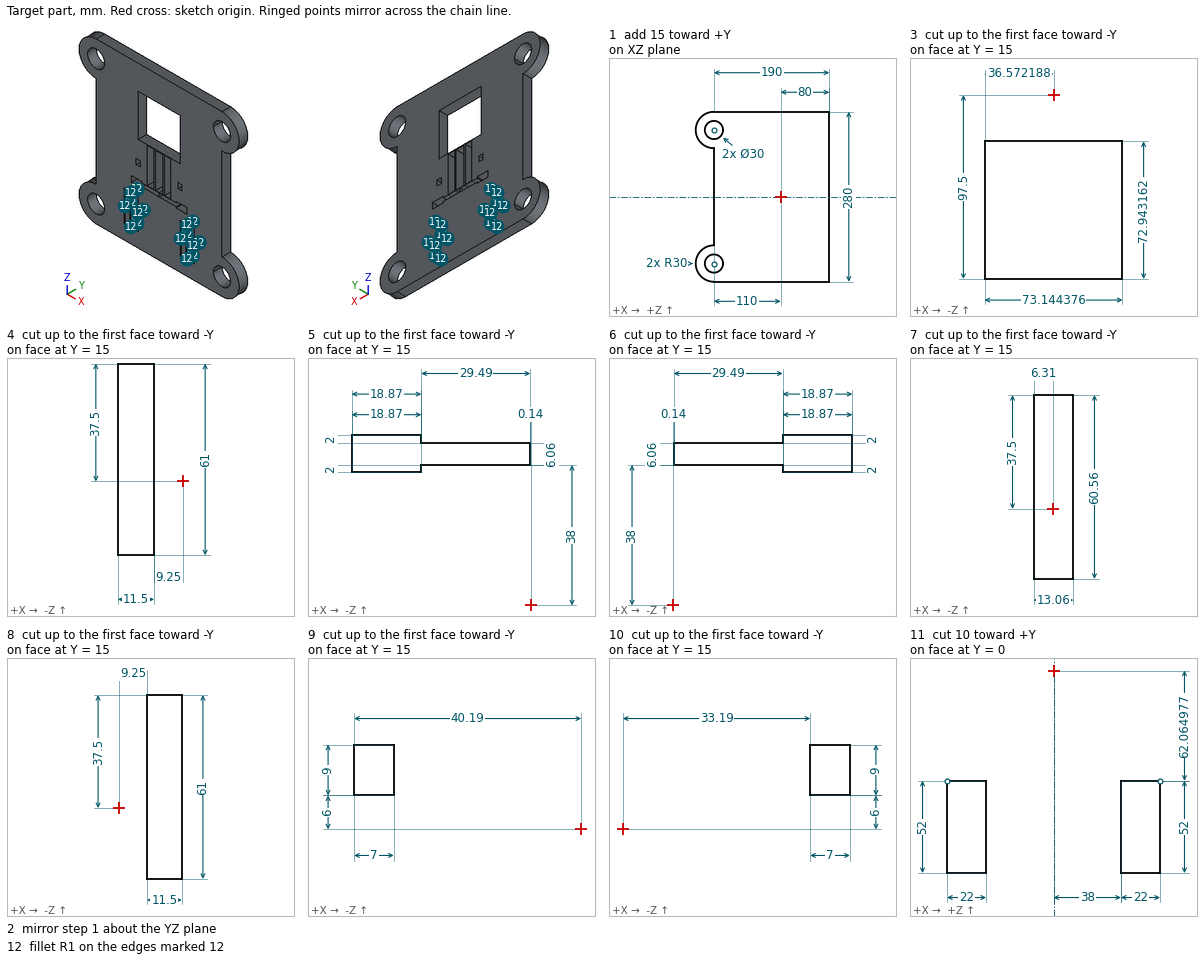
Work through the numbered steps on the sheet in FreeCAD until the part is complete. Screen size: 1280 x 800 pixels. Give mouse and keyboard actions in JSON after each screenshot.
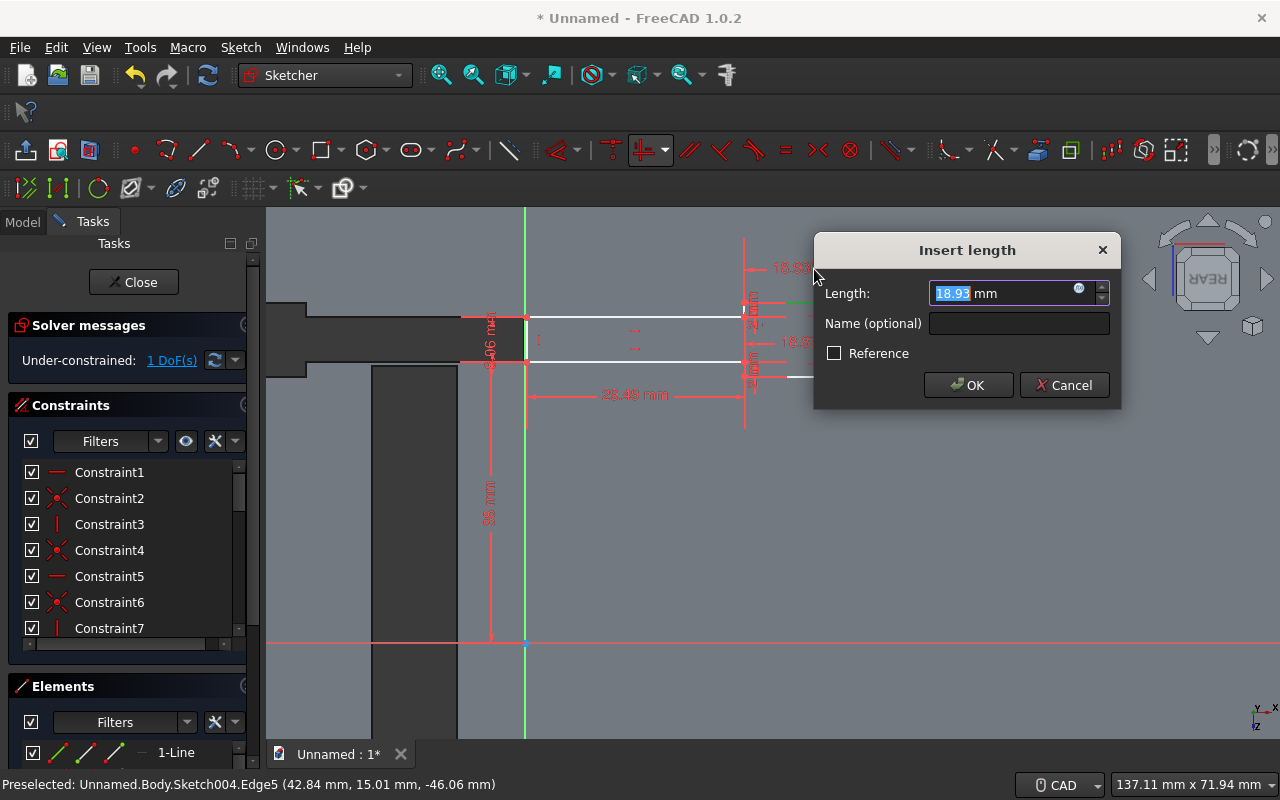
{"action": "type", "text": "18.87"}
{"action": "key", "text": "Return"}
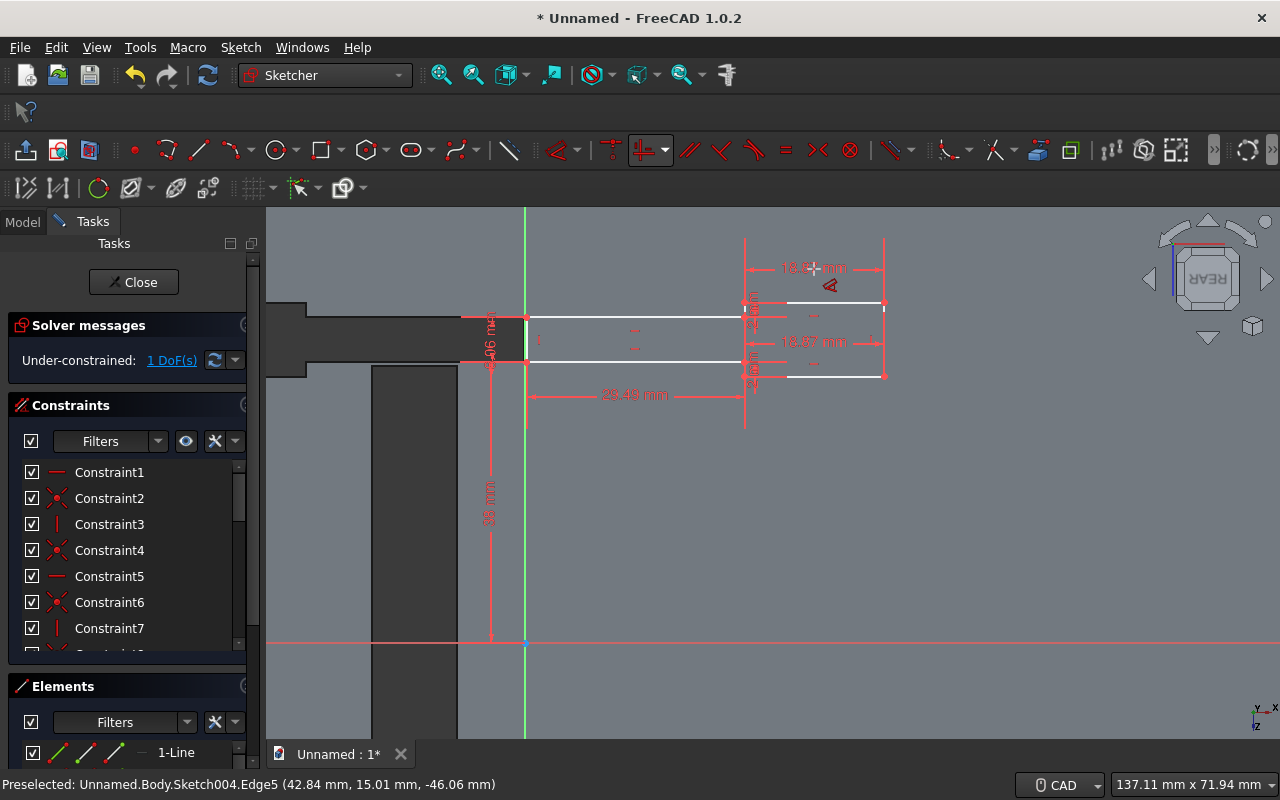
{"action": "scroll", "coordinate": [527, 362], "scroll_direction": "up", "scroll_amount": 19}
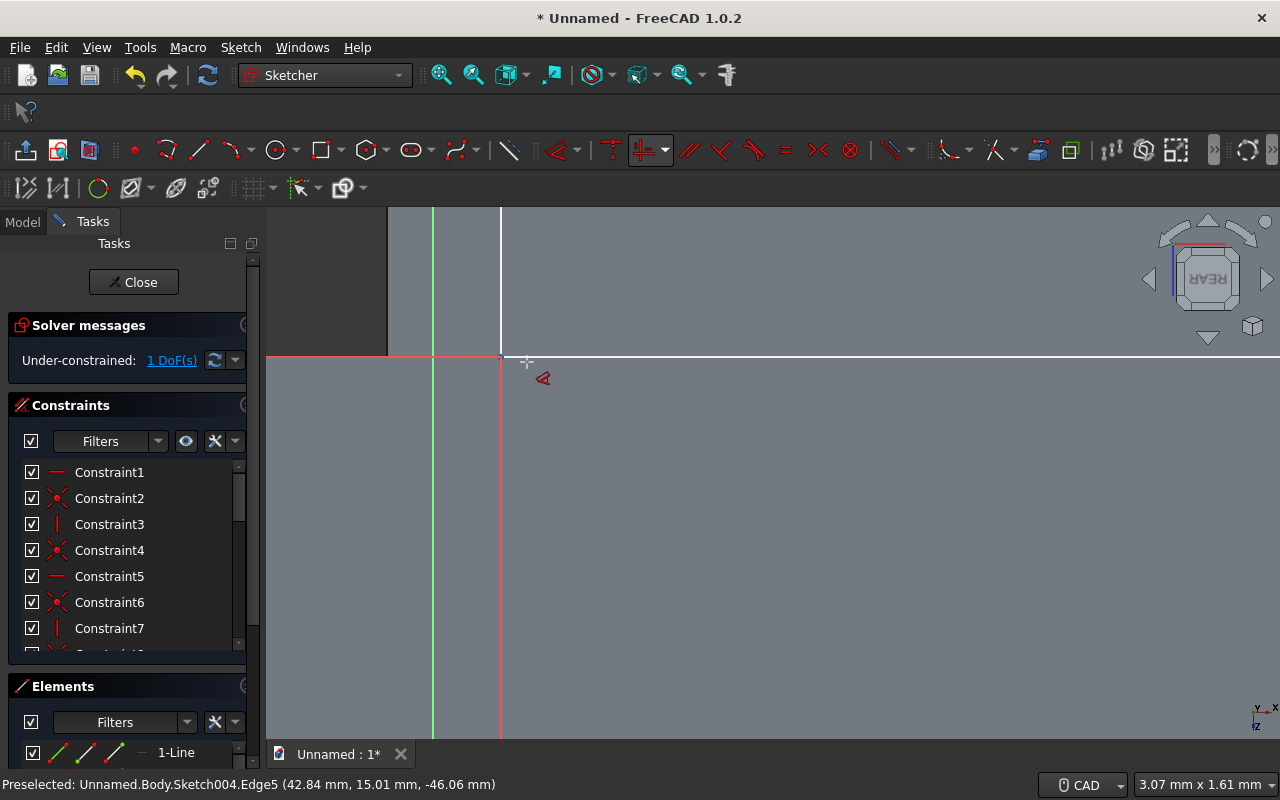
{"action": "left_click", "coordinate": [501, 357]}
{"action": "left_click", "coordinate": [467, 323]}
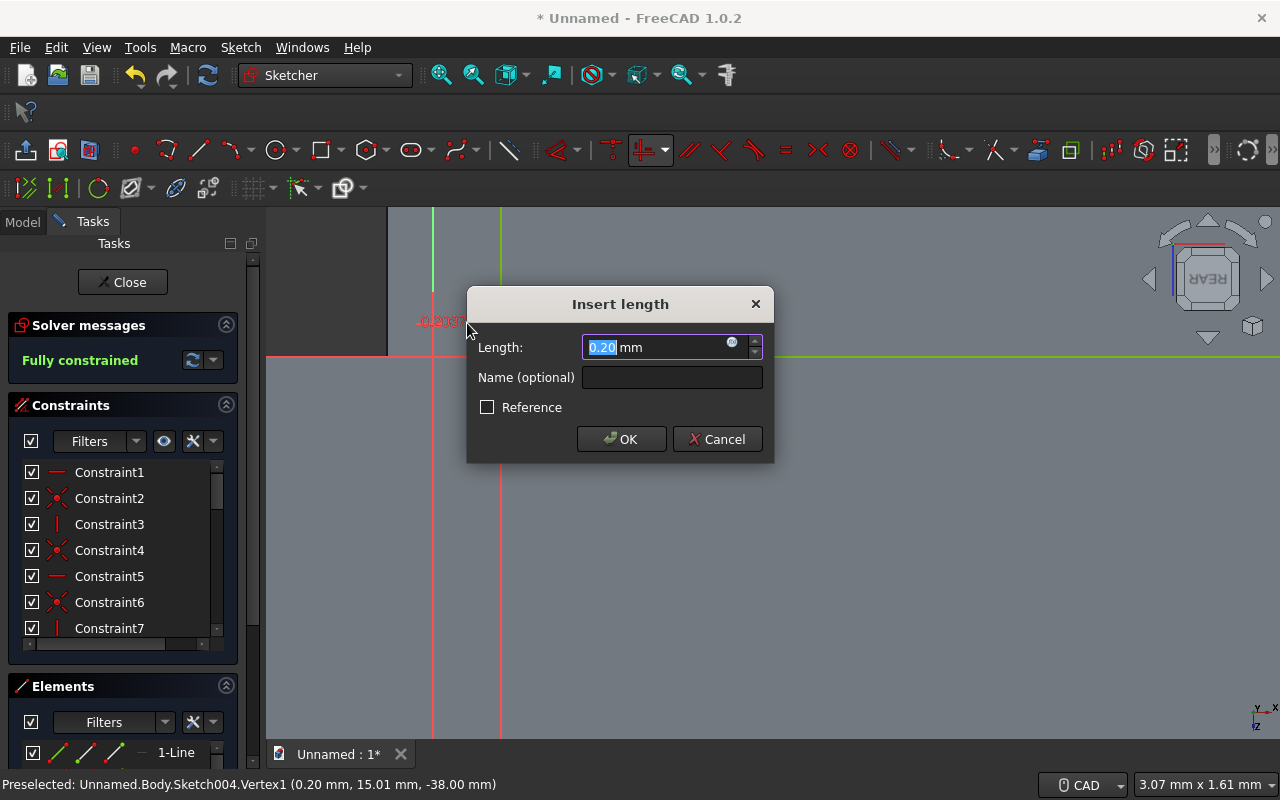
{"action": "type", "text": "0.14"}
{"action": "key", "text": "Return"}
{"action": "key", "text": "Escape"}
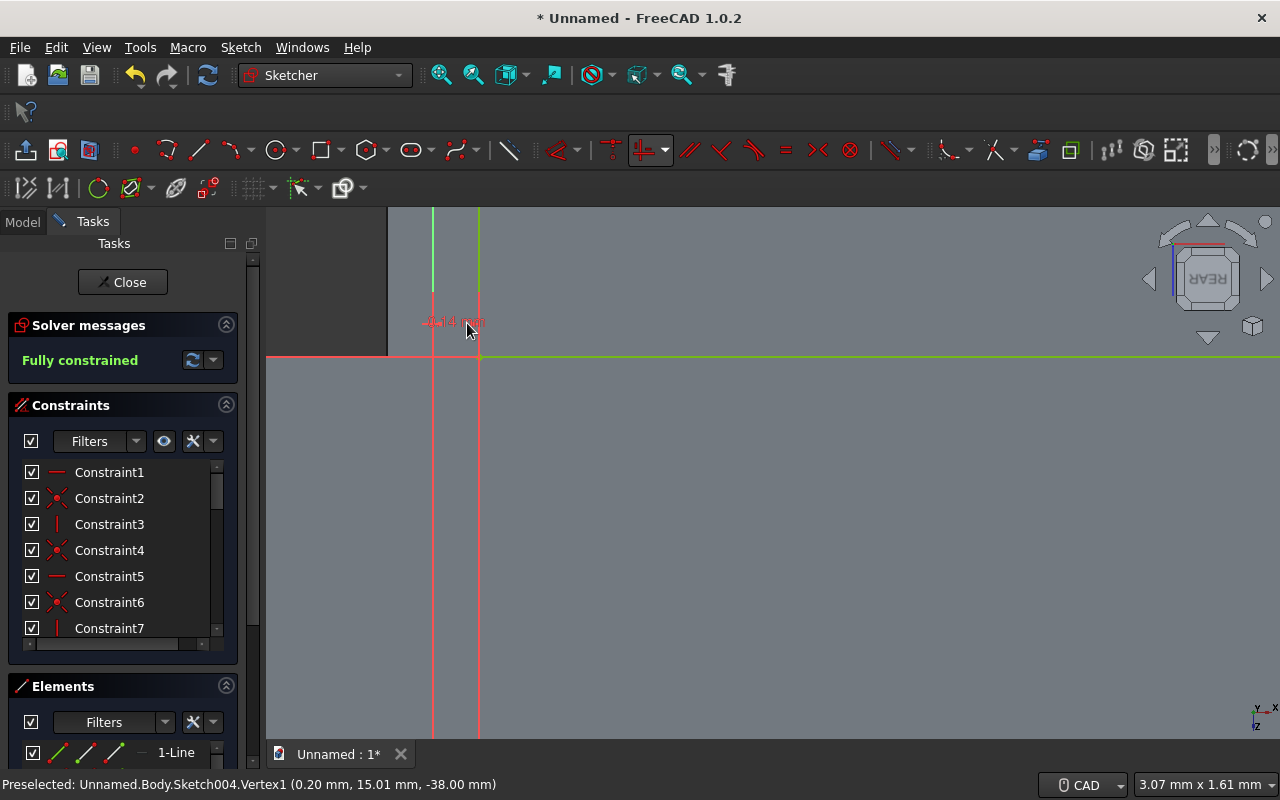
{"action": "left_click", "coordinate": [123, 282]}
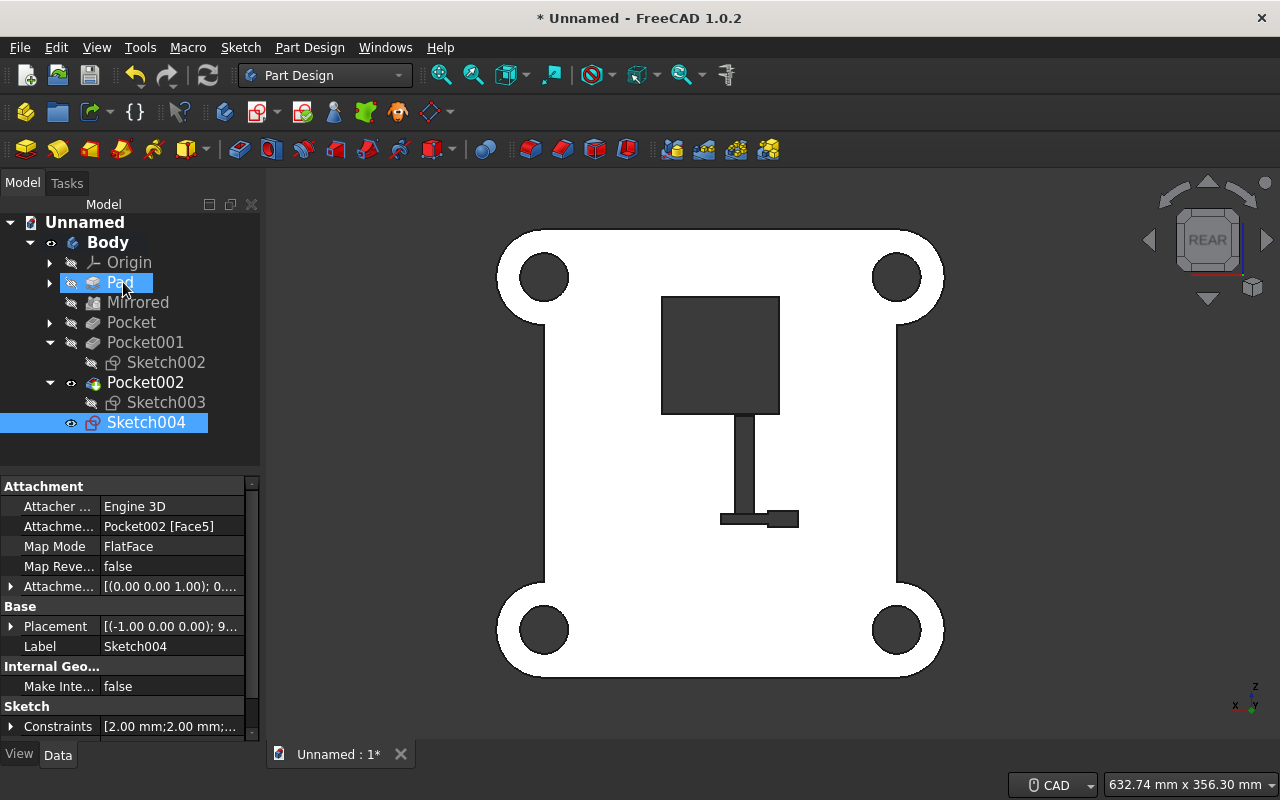
{"action": "left_click", "coordinate": [240, 150]}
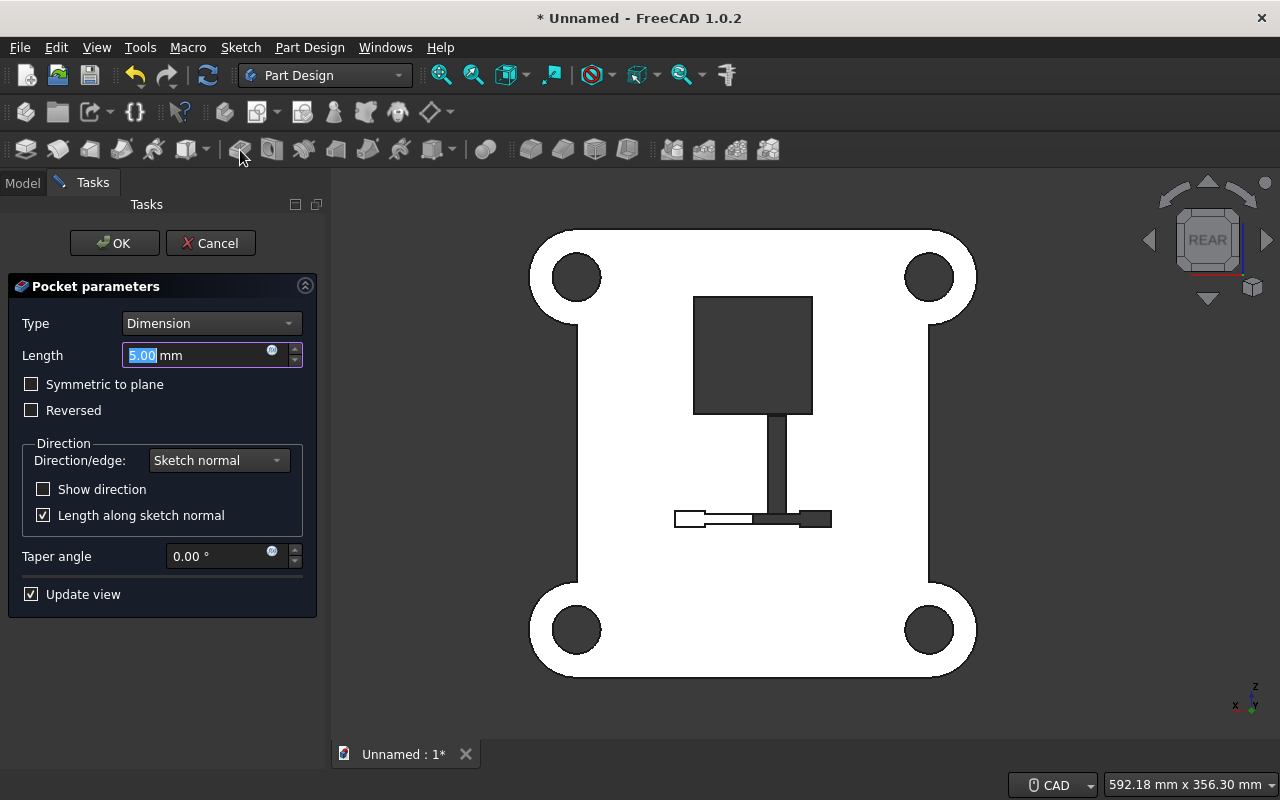
{"action": "left_click", "coordinate": [212, 324]}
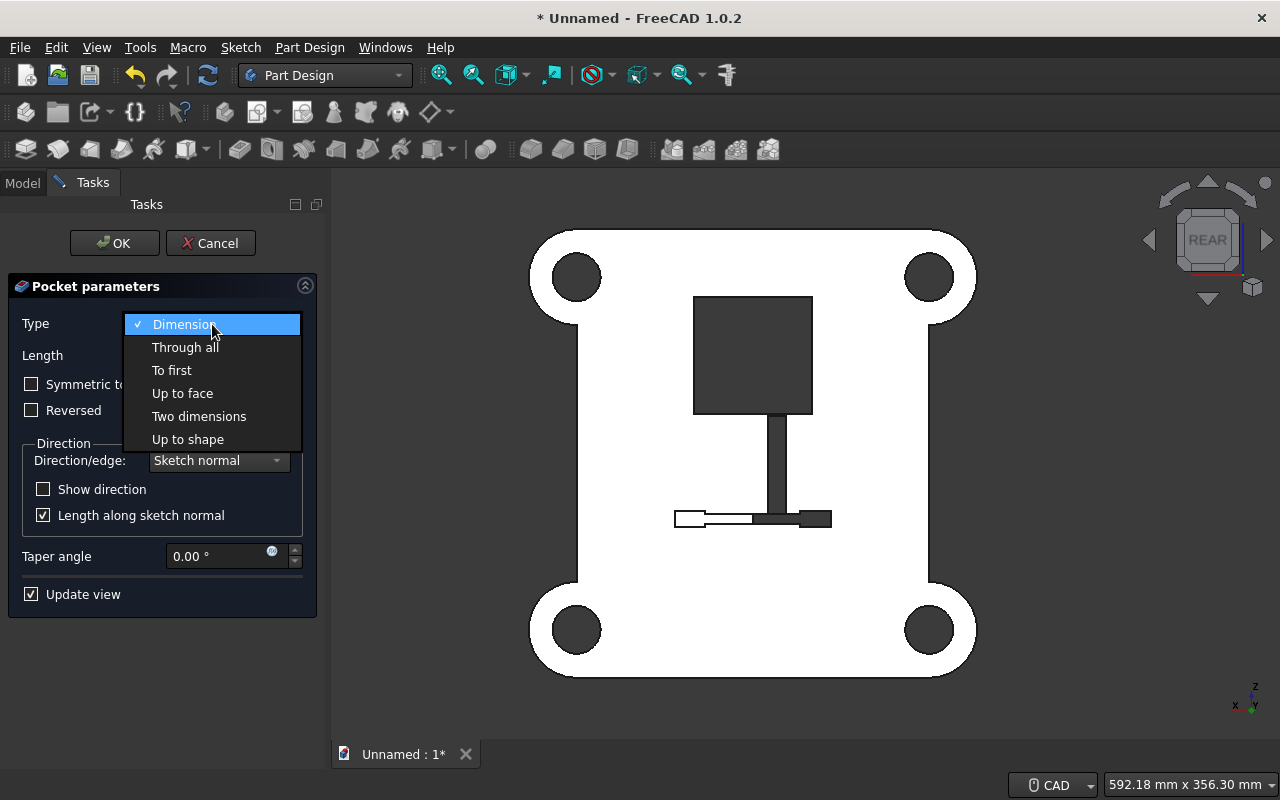
{"action": "left_click", "coordinate": [212, 370]}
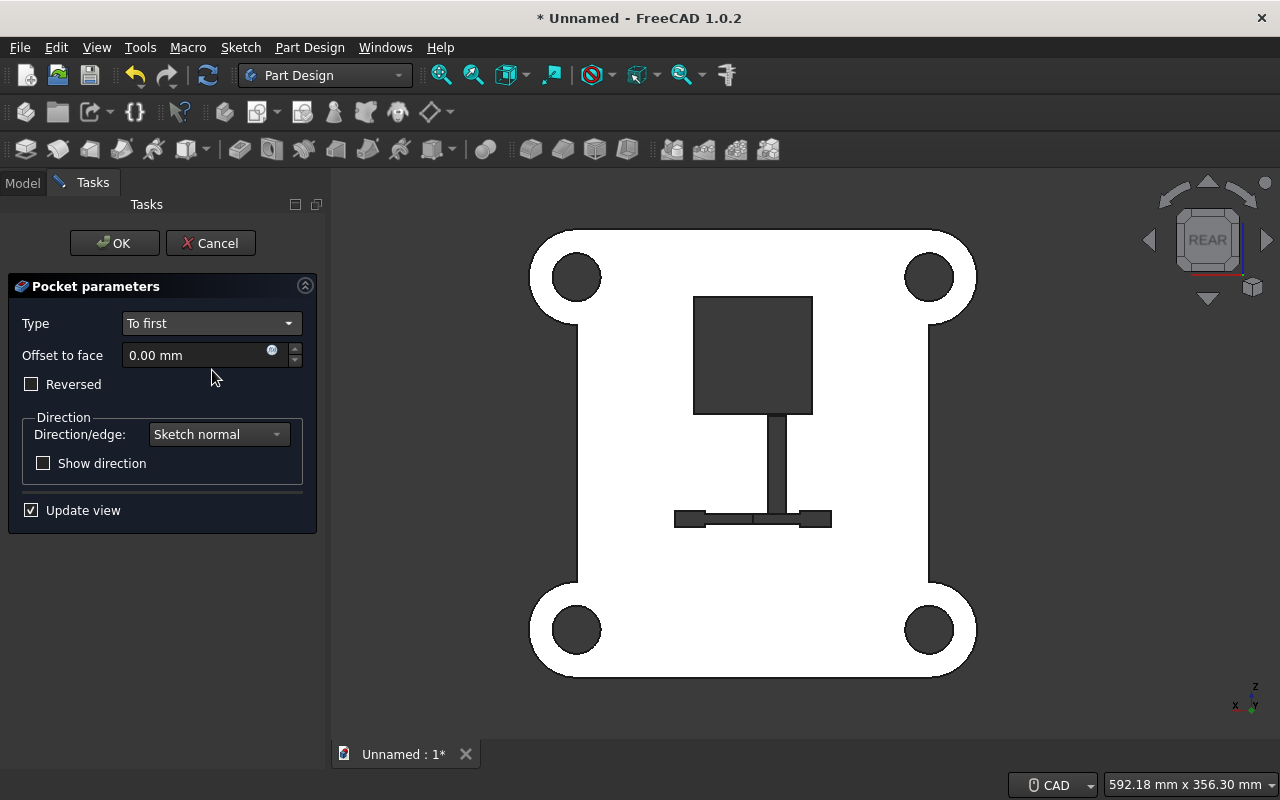
{"action": "left_click", "coordinate": [115, 243]}